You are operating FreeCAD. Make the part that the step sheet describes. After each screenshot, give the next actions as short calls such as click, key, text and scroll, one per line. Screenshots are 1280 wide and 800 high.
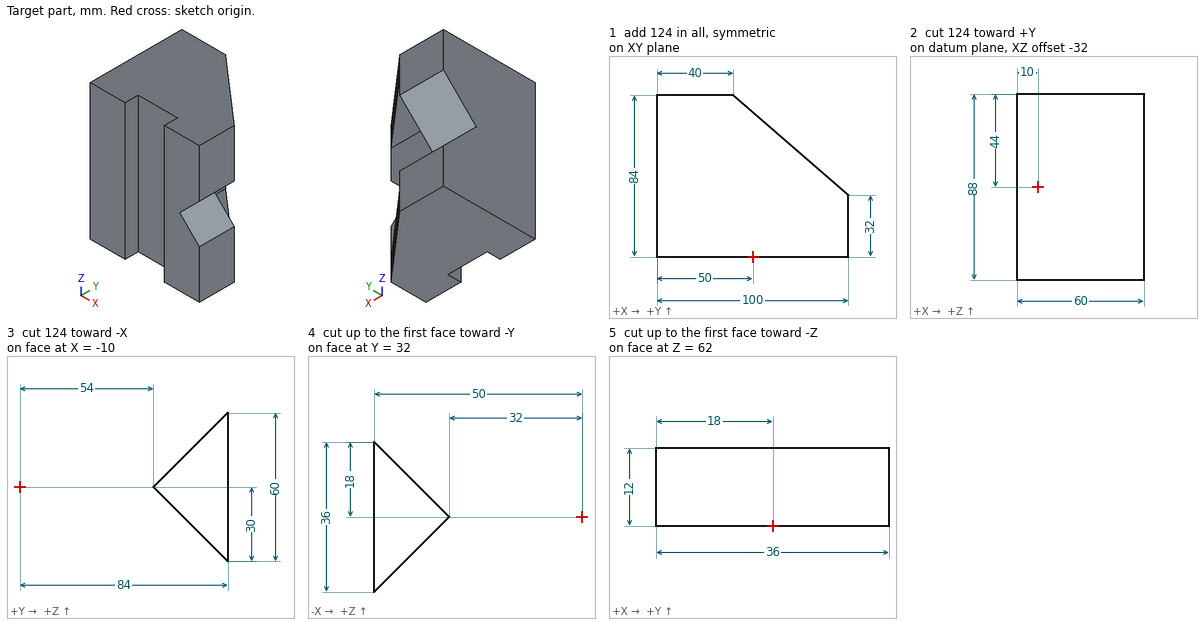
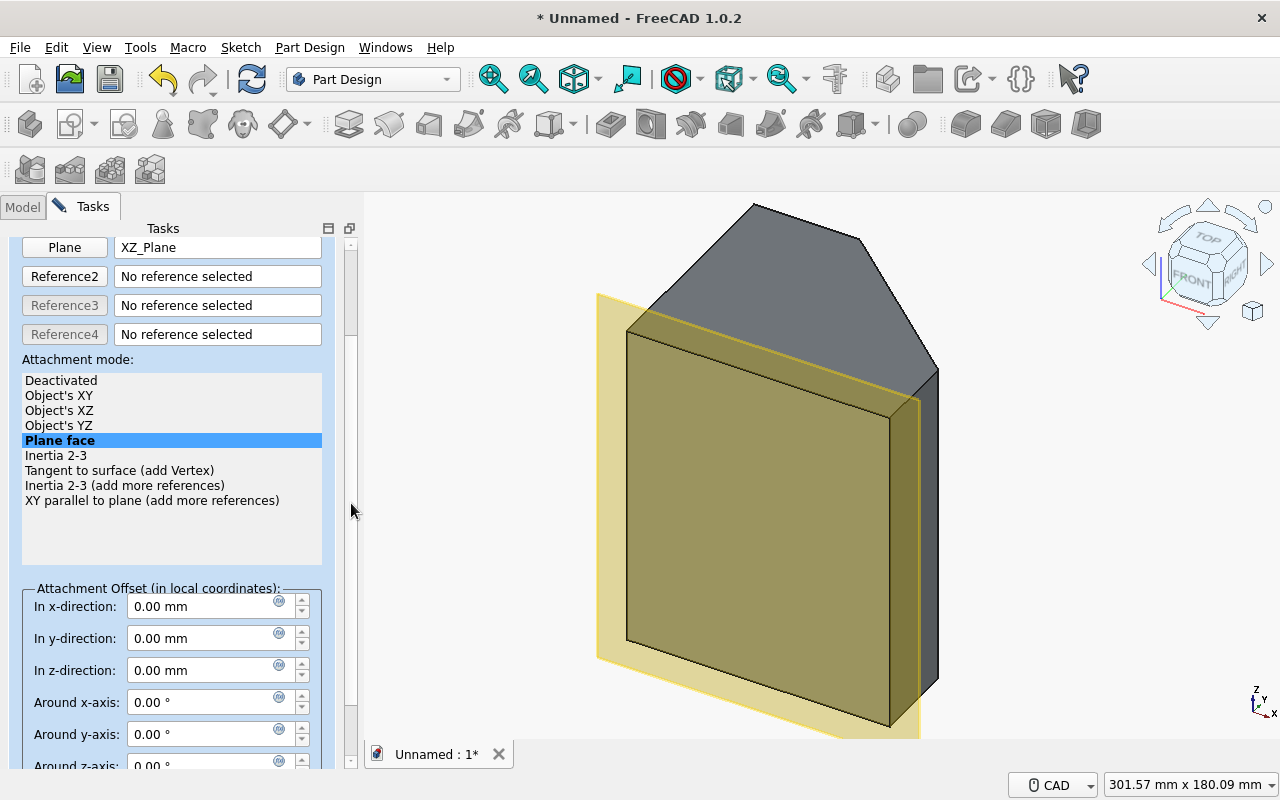
triple_click(210, 670)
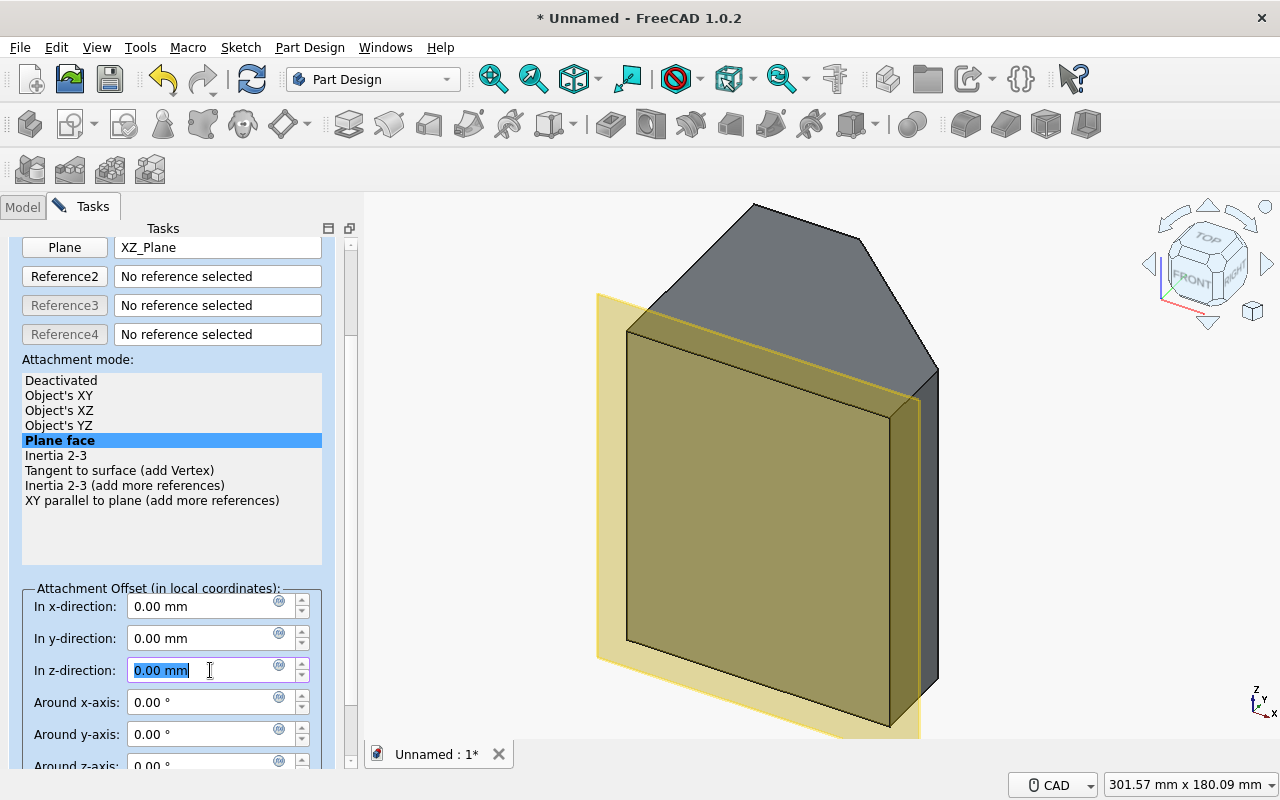
text(-32)
key(Tab)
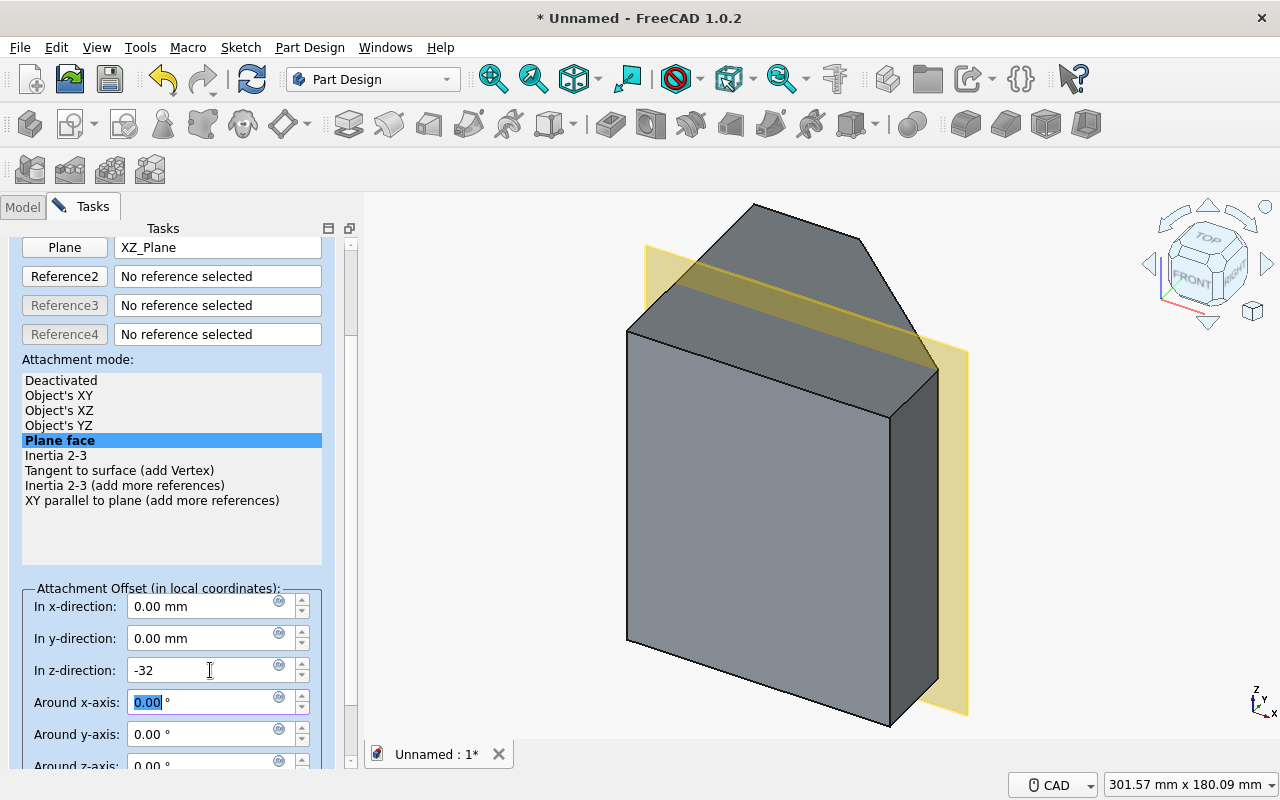
scroll(351, 503, up, 3)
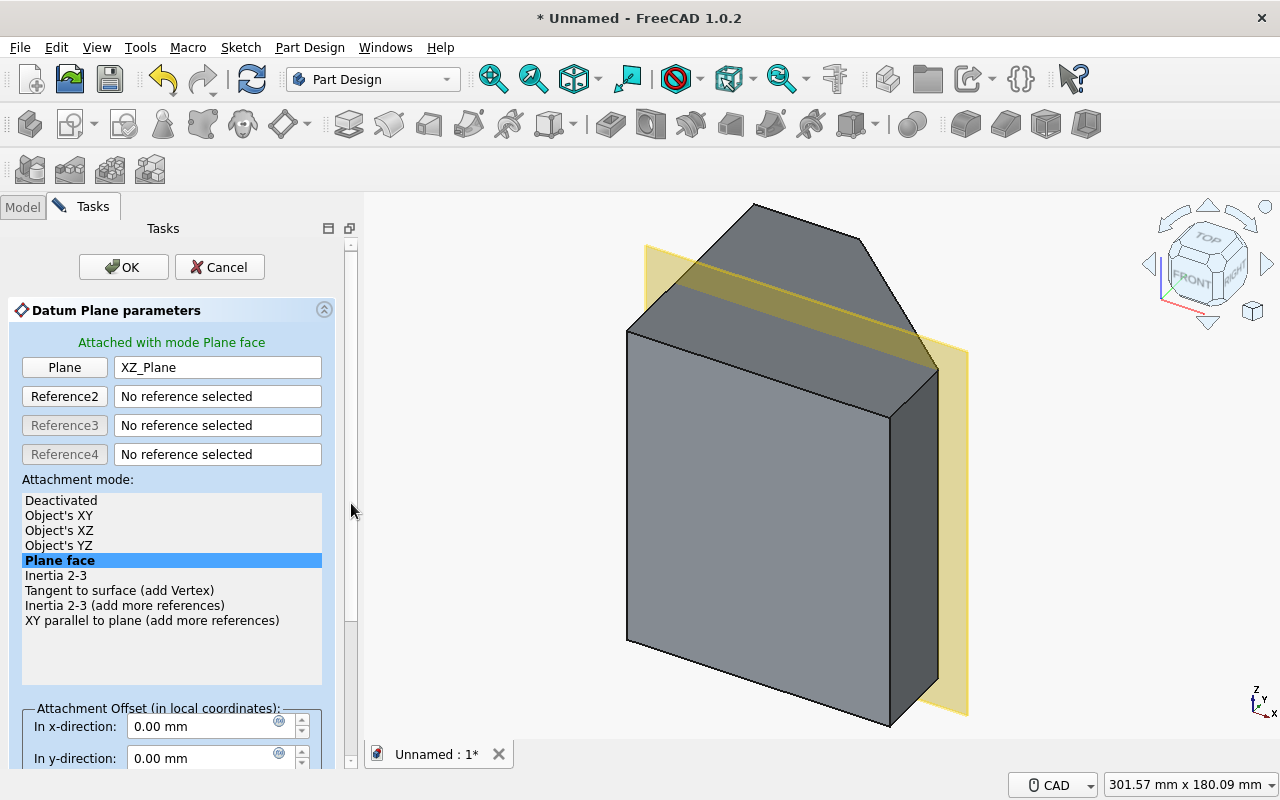
click(124, 267)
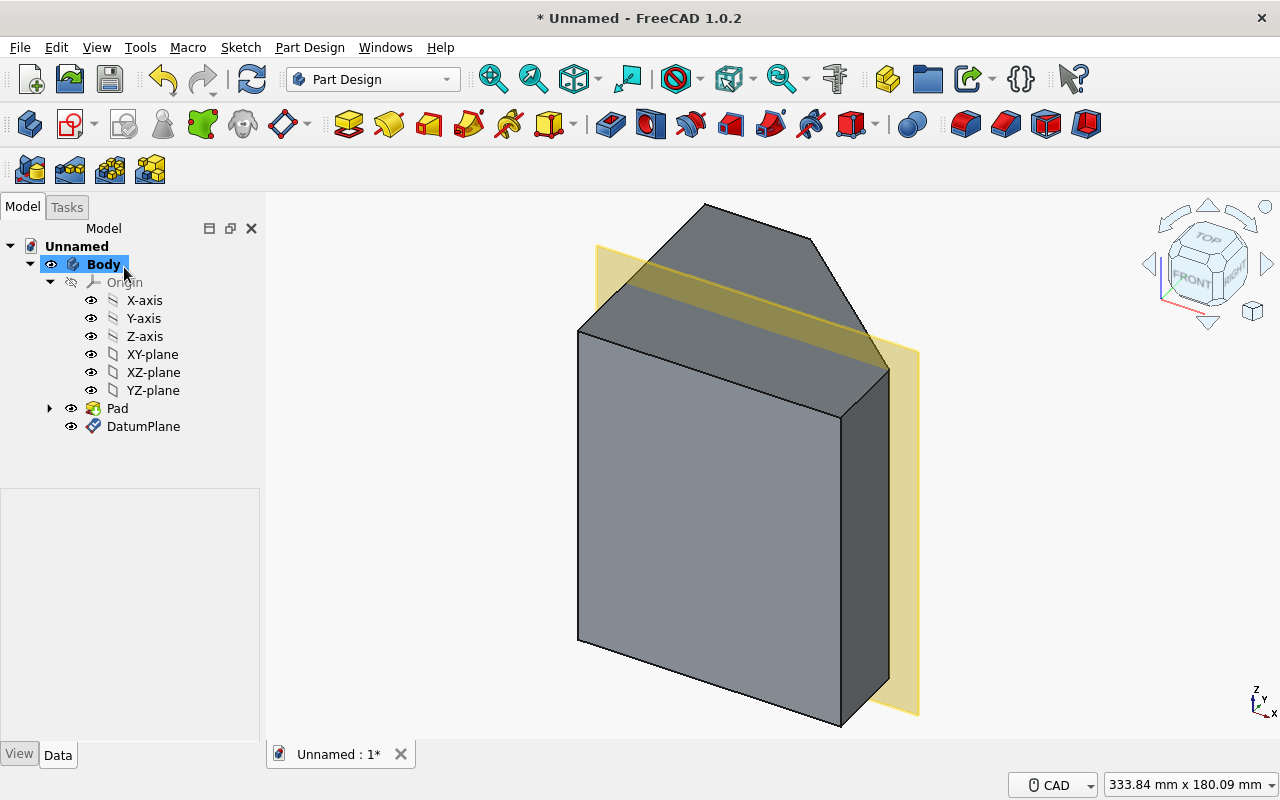
click(116, 426)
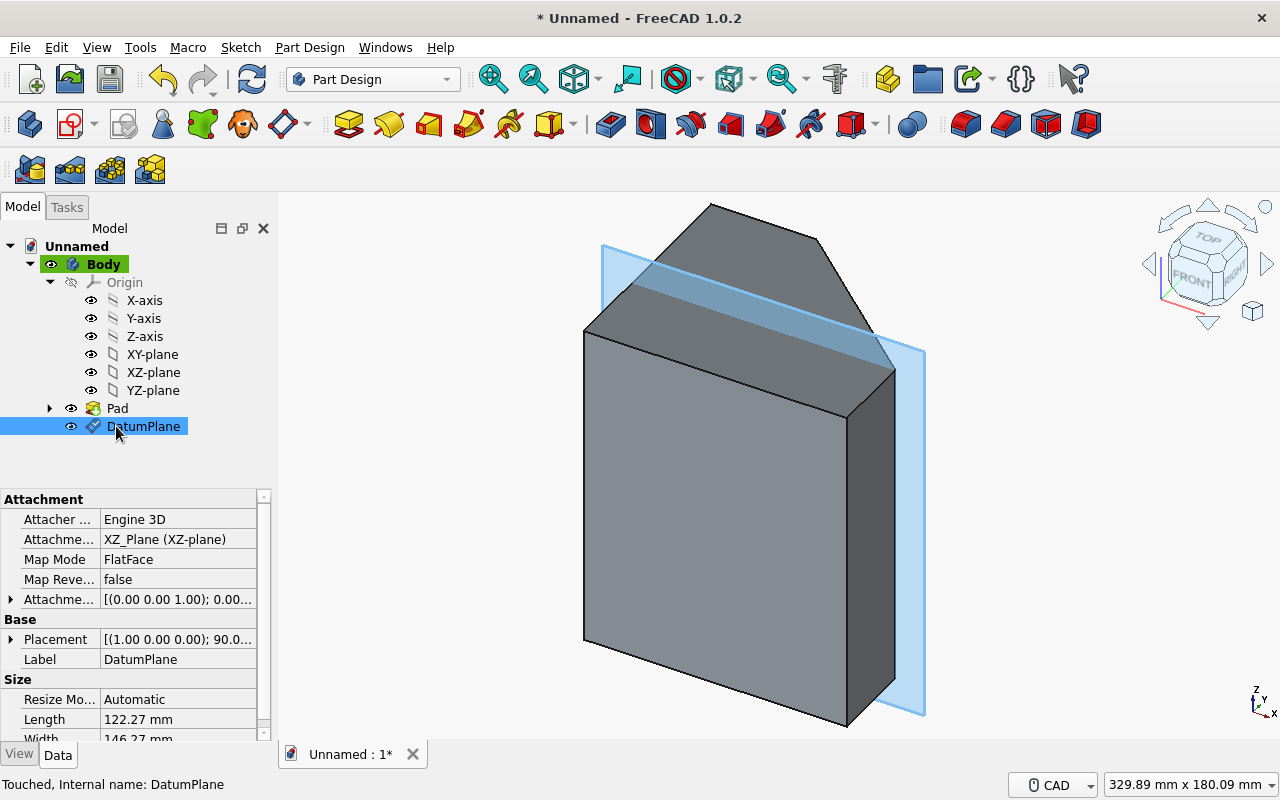
click(70, 124)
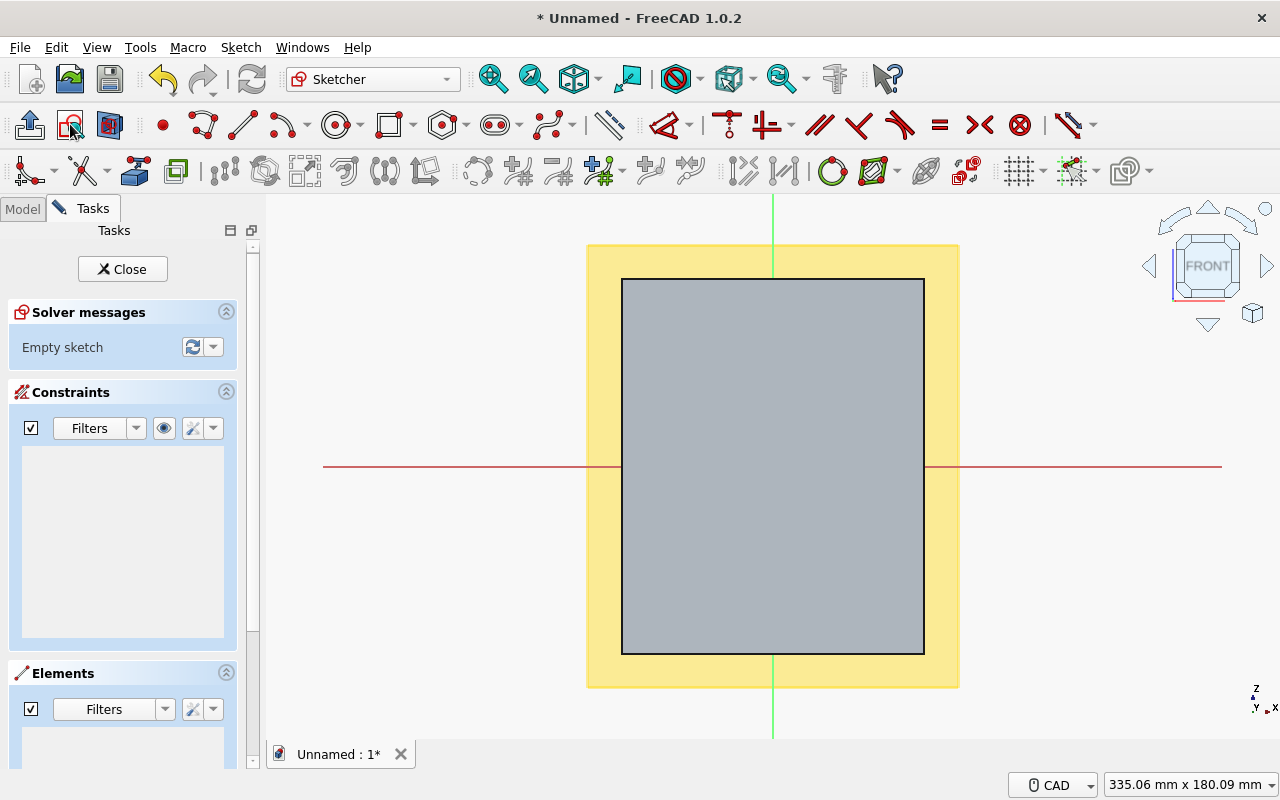
click(110, 126)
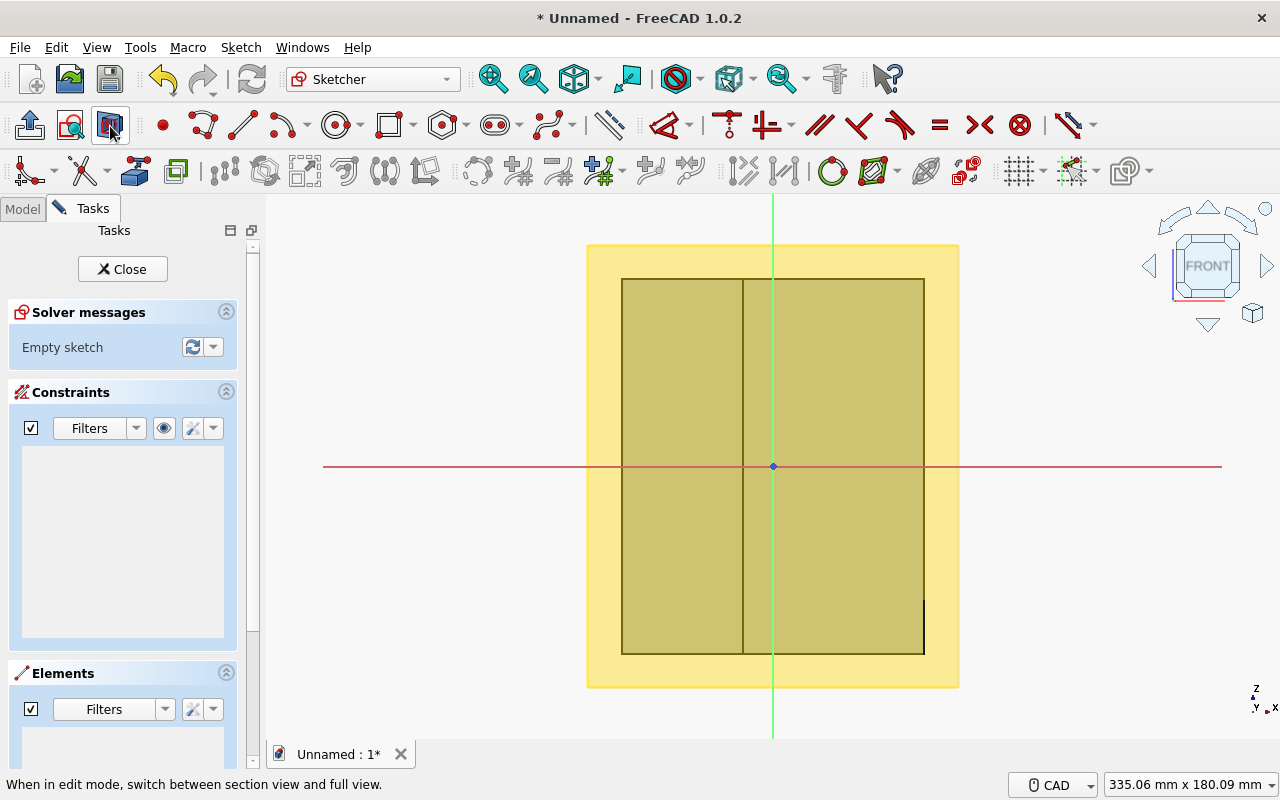
click(390, 126)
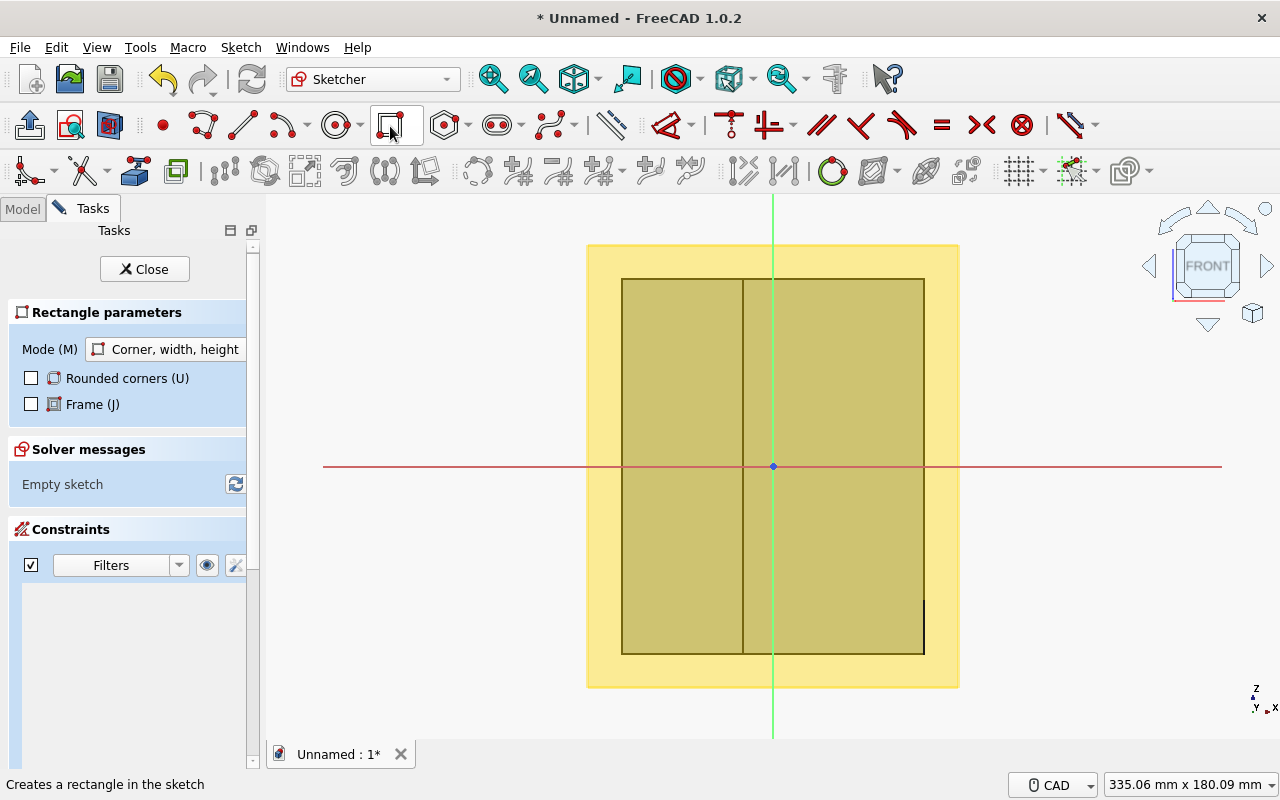
click(743, 333)
click(924, 600)
key(Escape)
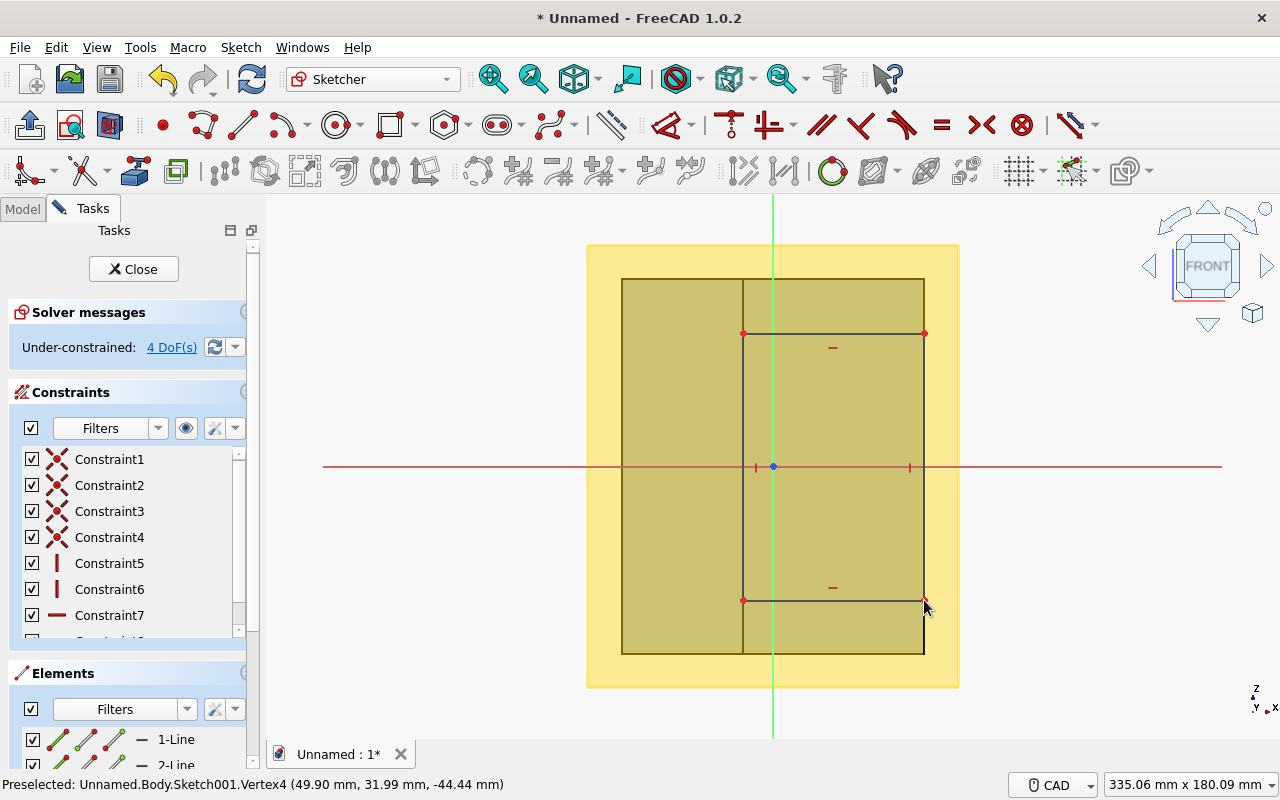
click(666, 126)